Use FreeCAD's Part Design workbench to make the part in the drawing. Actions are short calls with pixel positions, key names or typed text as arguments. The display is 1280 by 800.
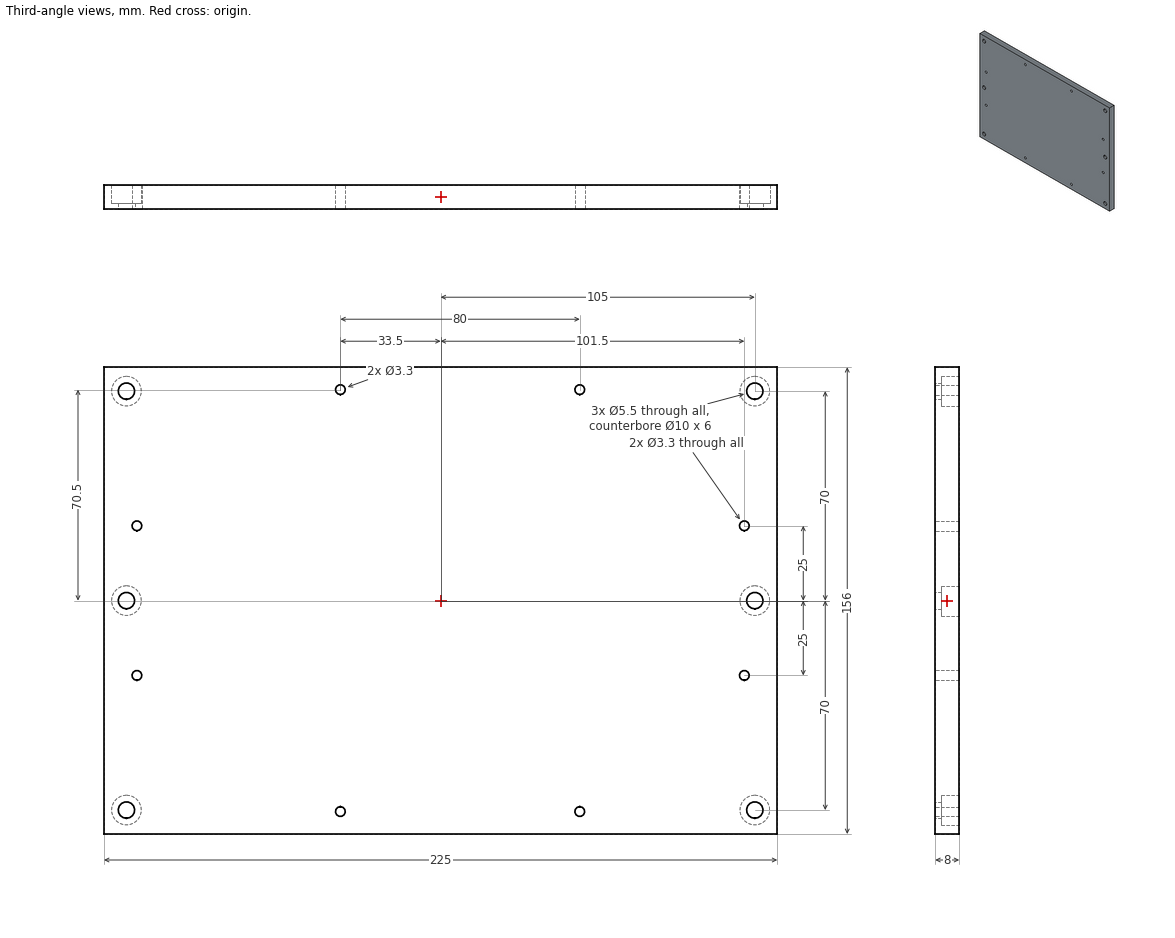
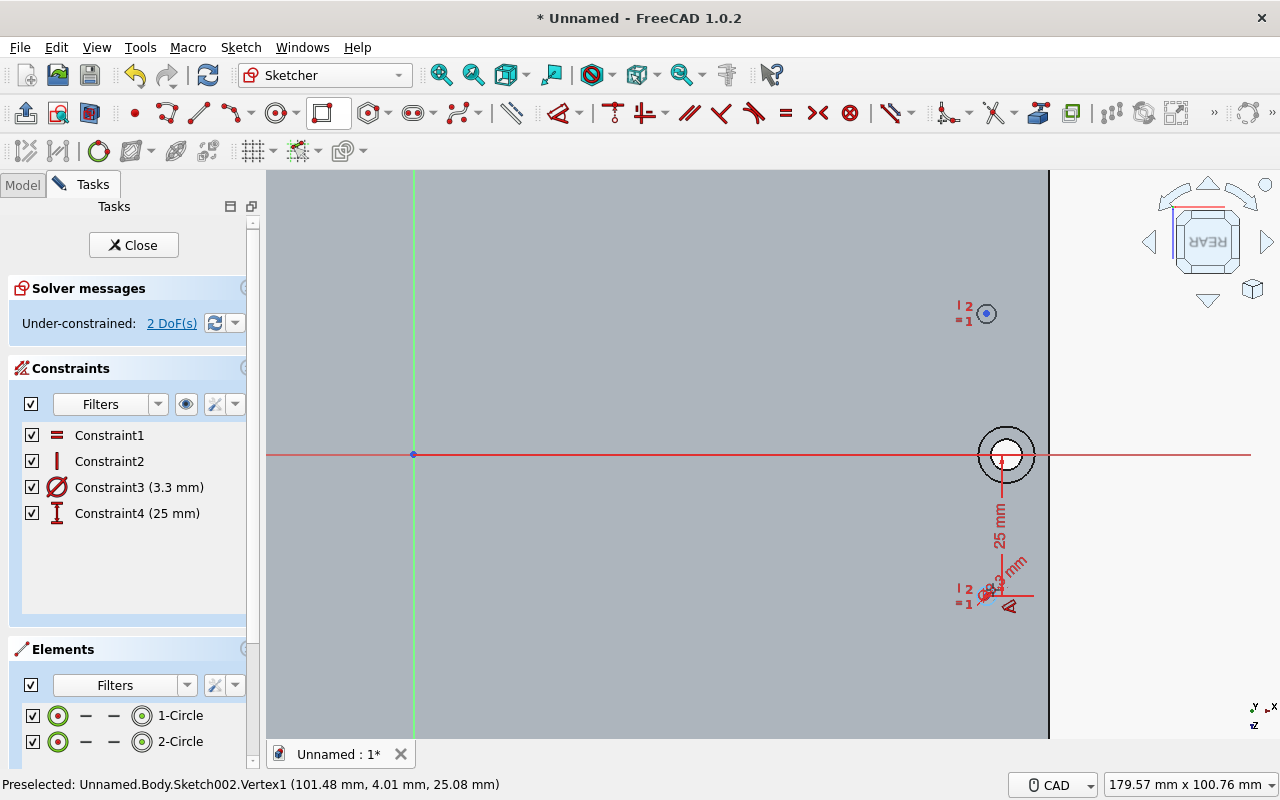
click(987, 314)
click(380, 384)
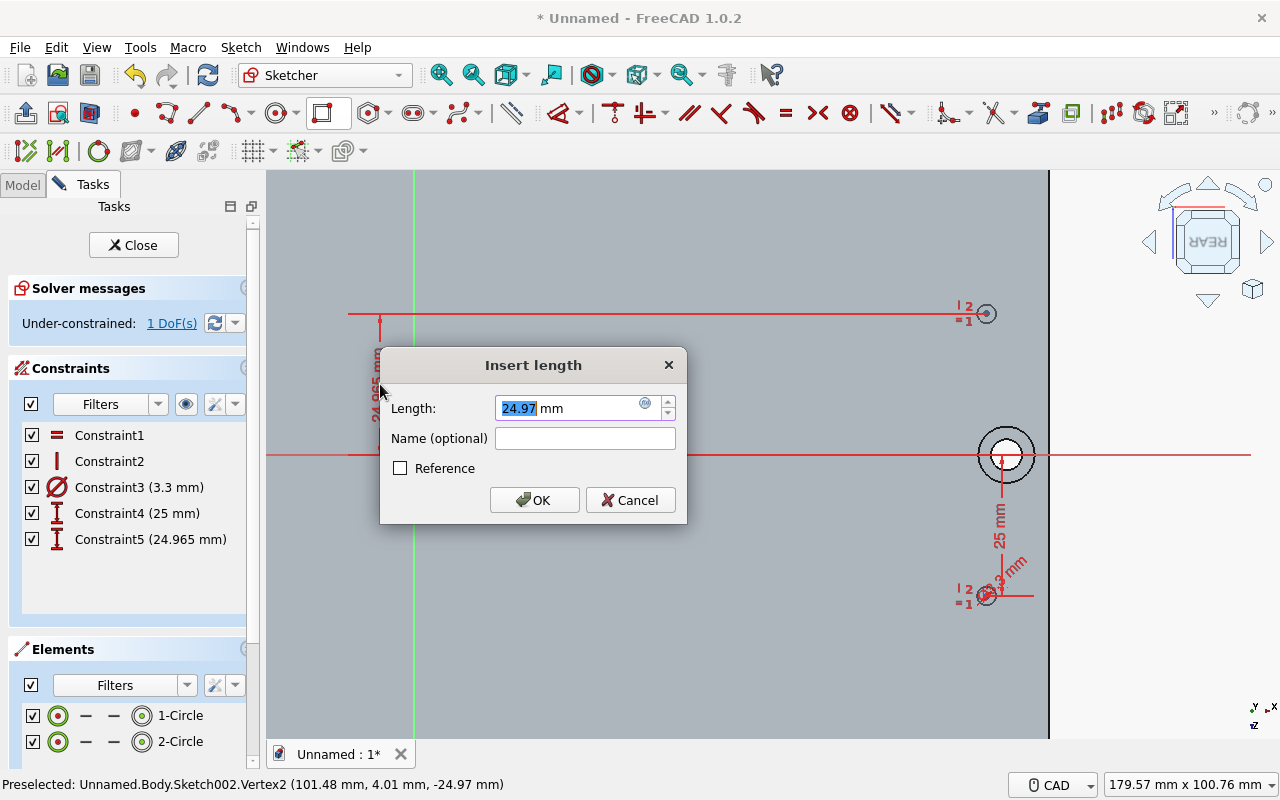
text(25)
key(Return)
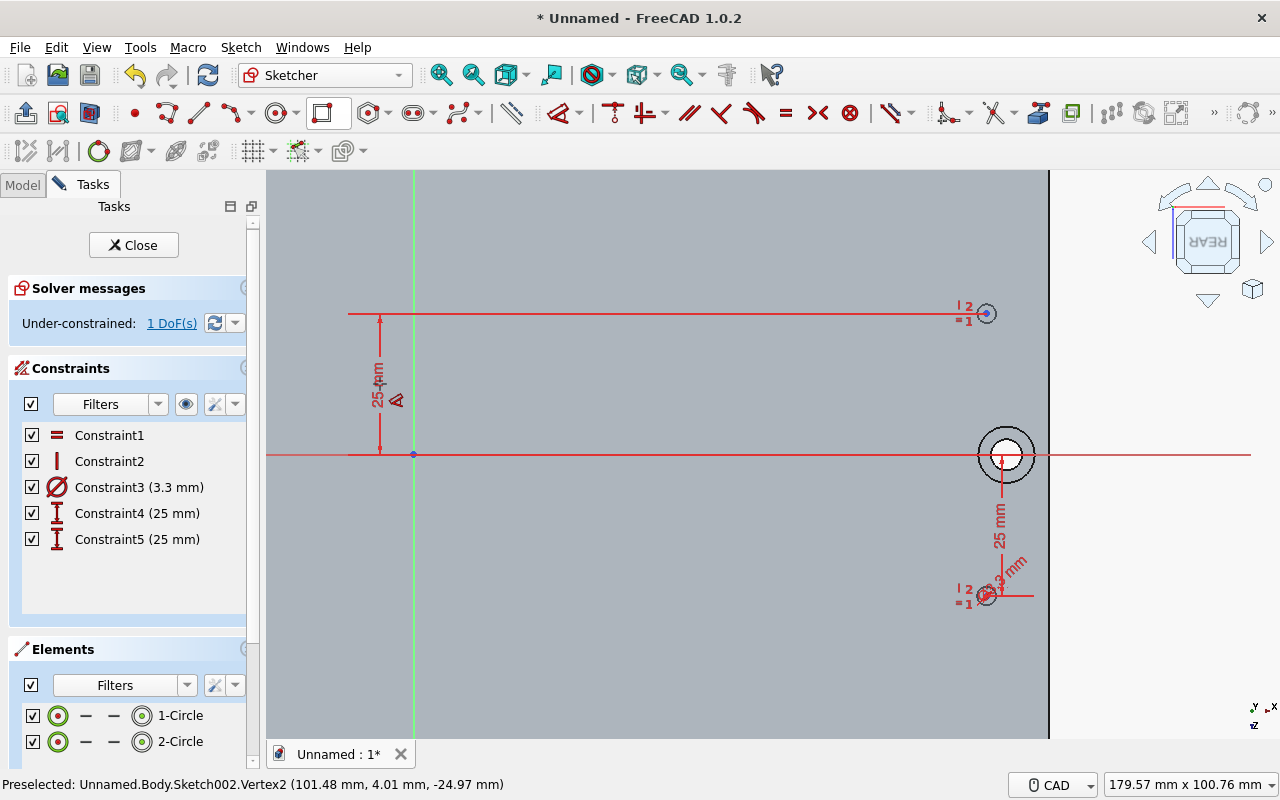
click(987, 596)
click(700, 630)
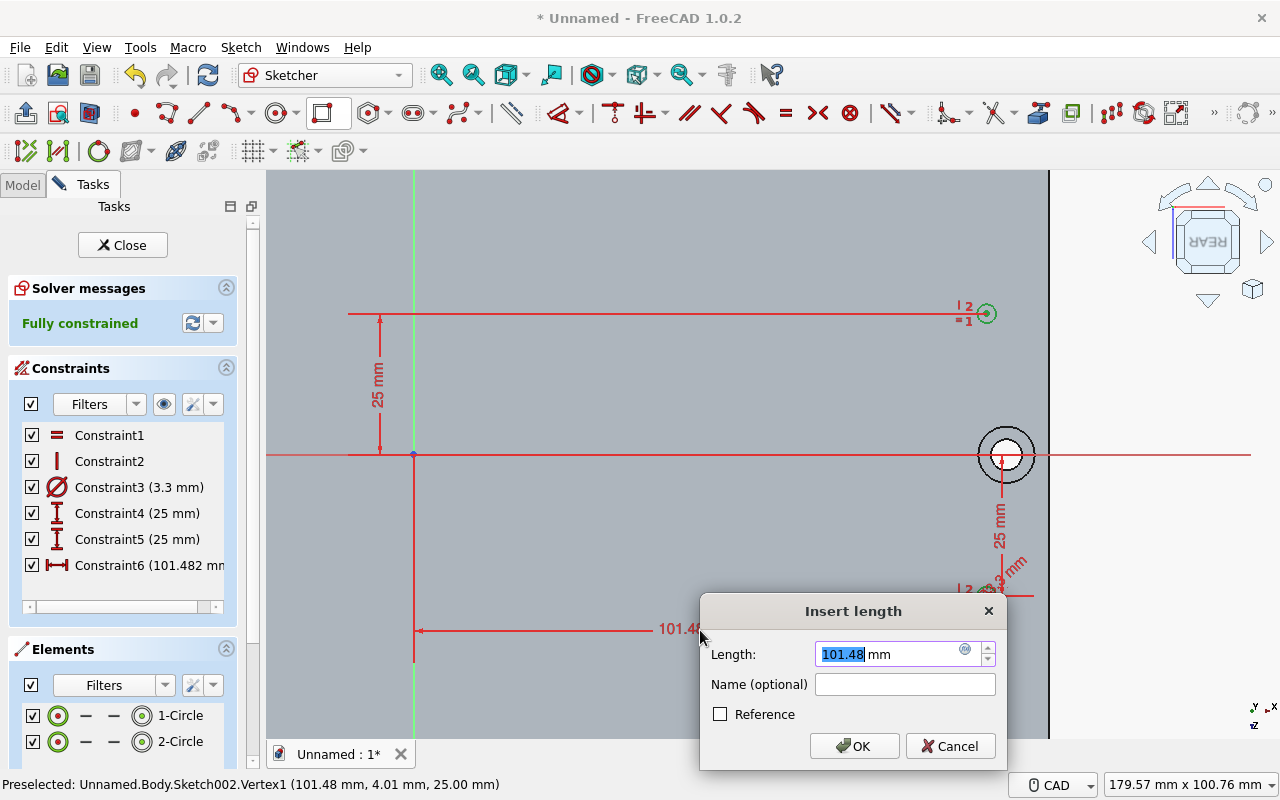
text(101.5)
key(Return)
key(Escape)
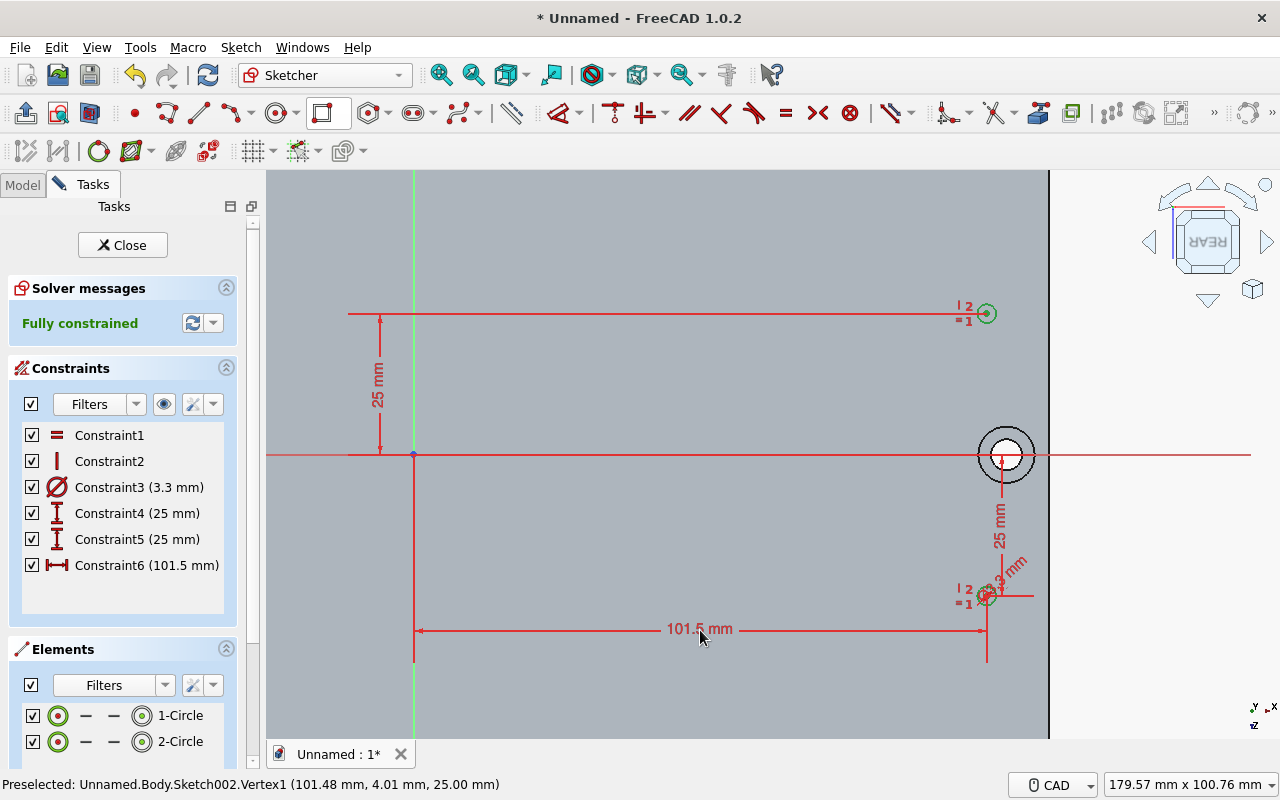
click(123, 245)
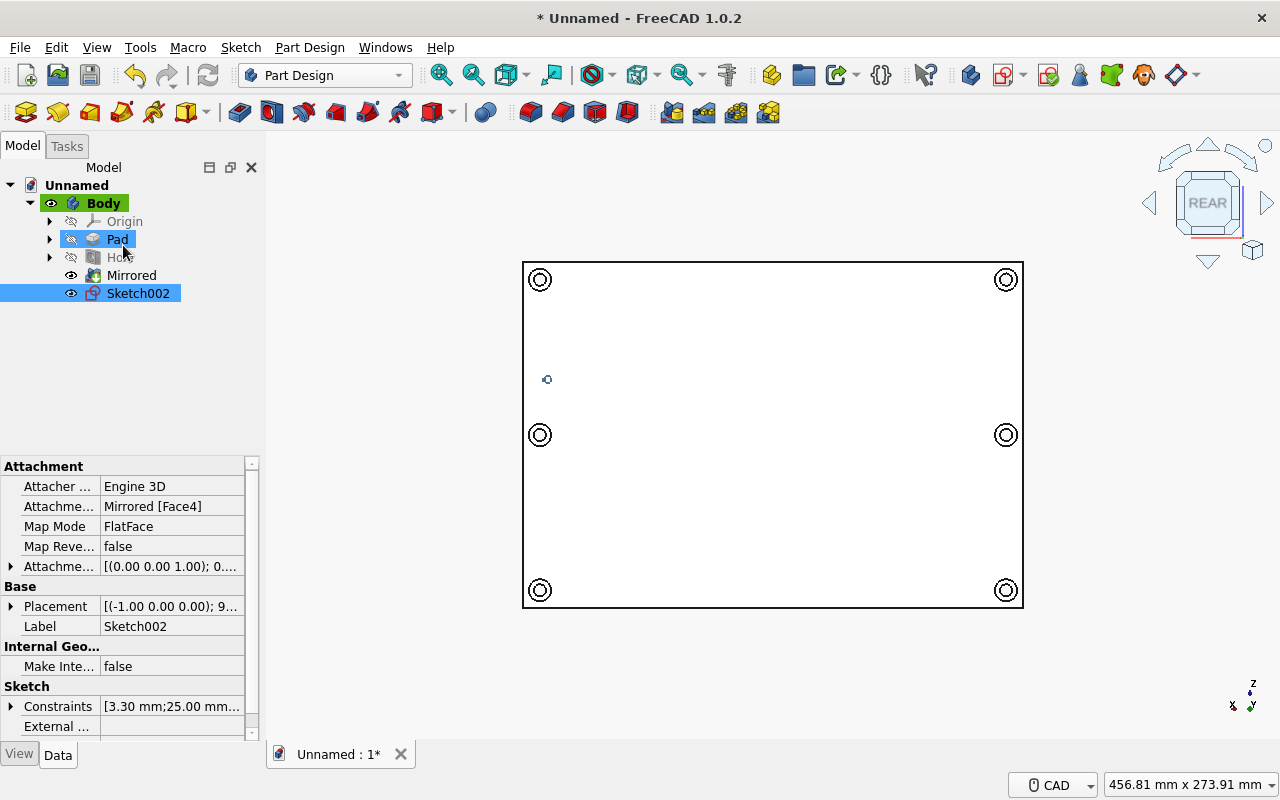
click(272, 112)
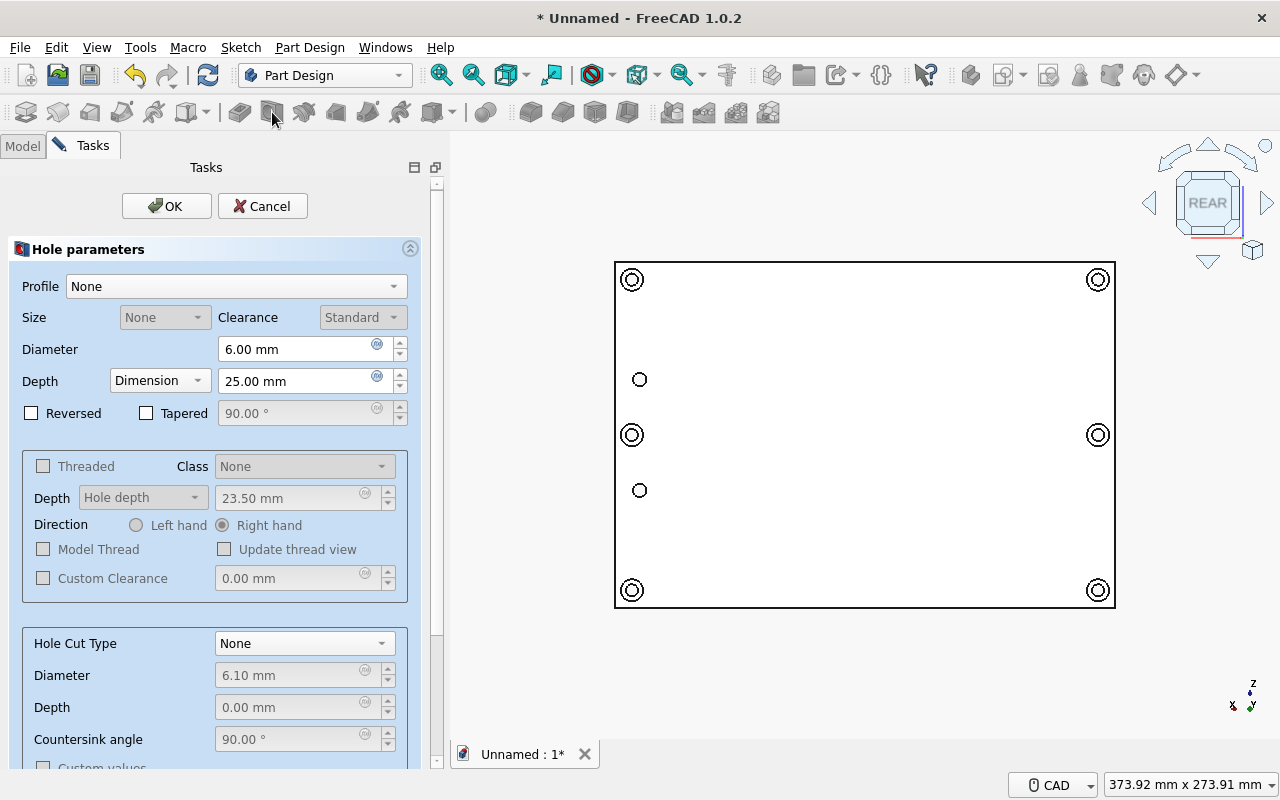
triple_click(305, 349)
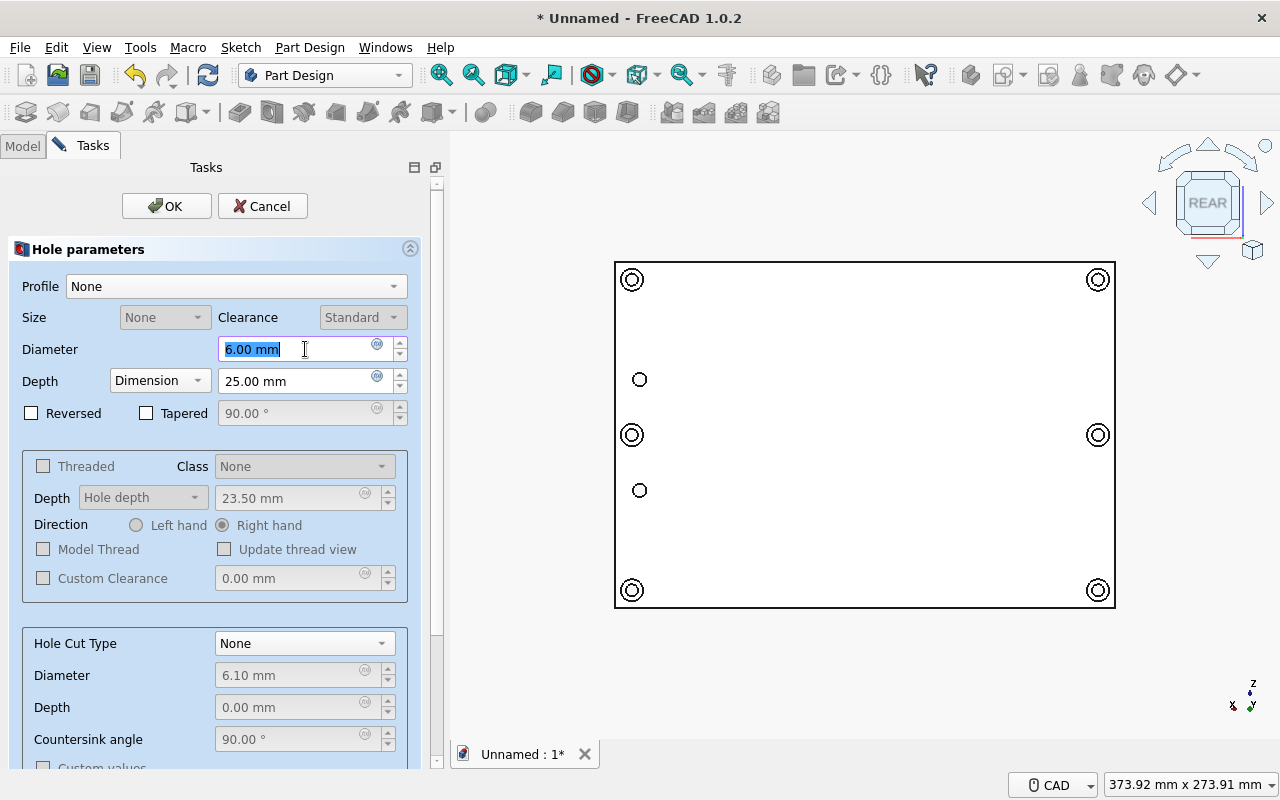
text(3.3)
key(Tab)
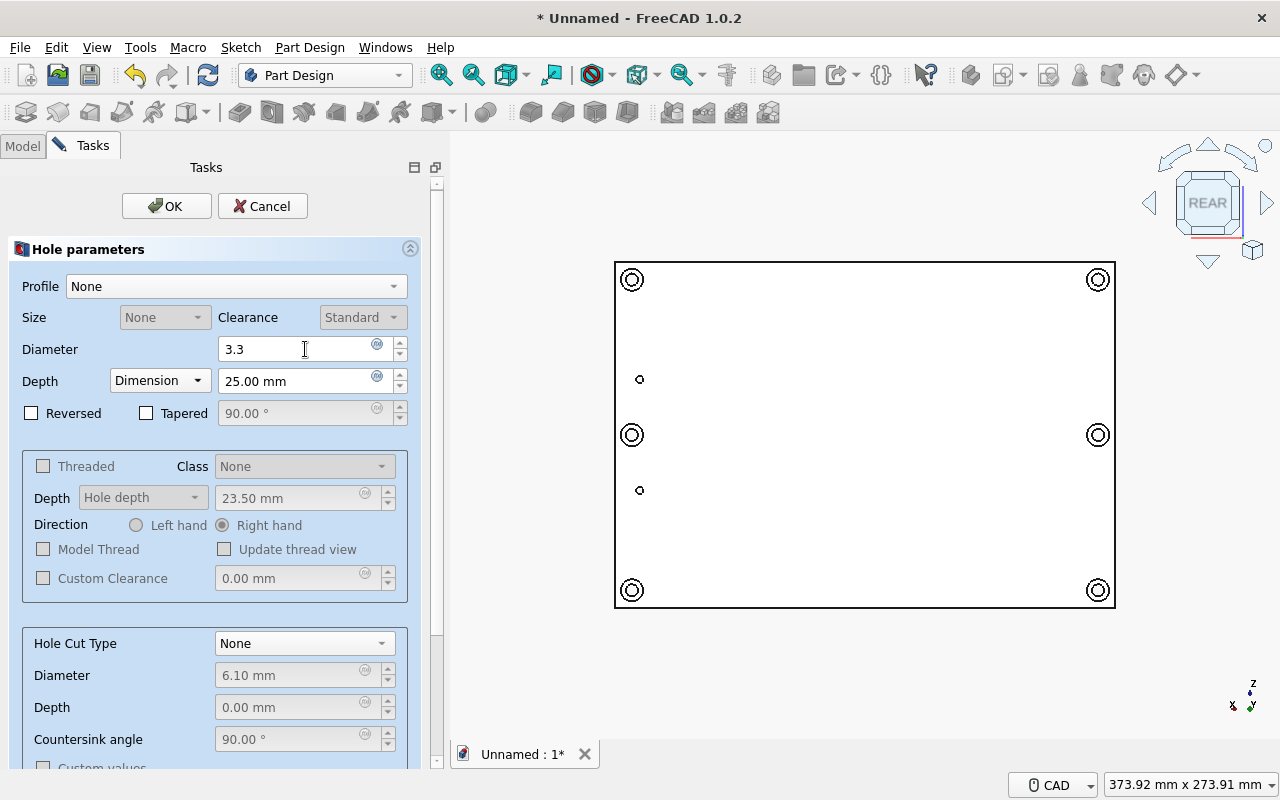
click(161, 380)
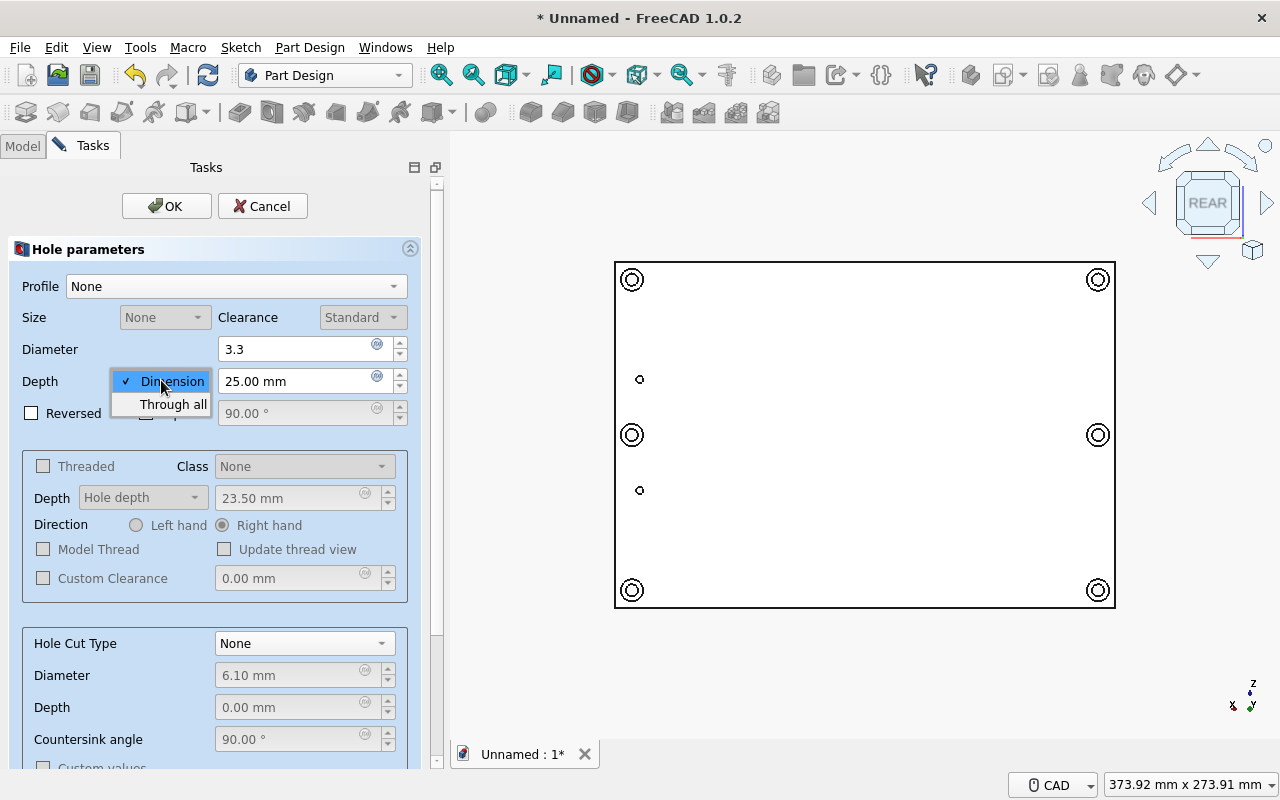
click(160, 404)